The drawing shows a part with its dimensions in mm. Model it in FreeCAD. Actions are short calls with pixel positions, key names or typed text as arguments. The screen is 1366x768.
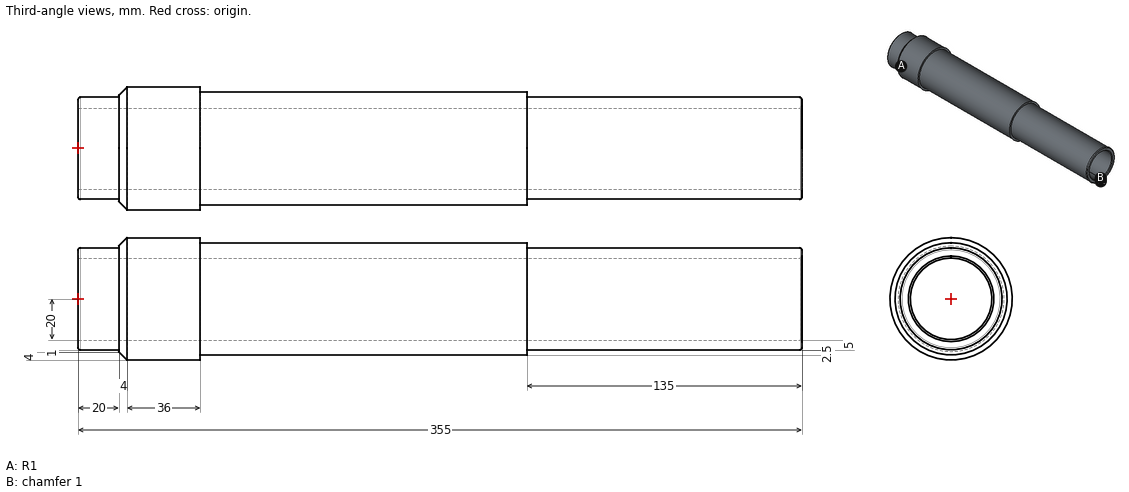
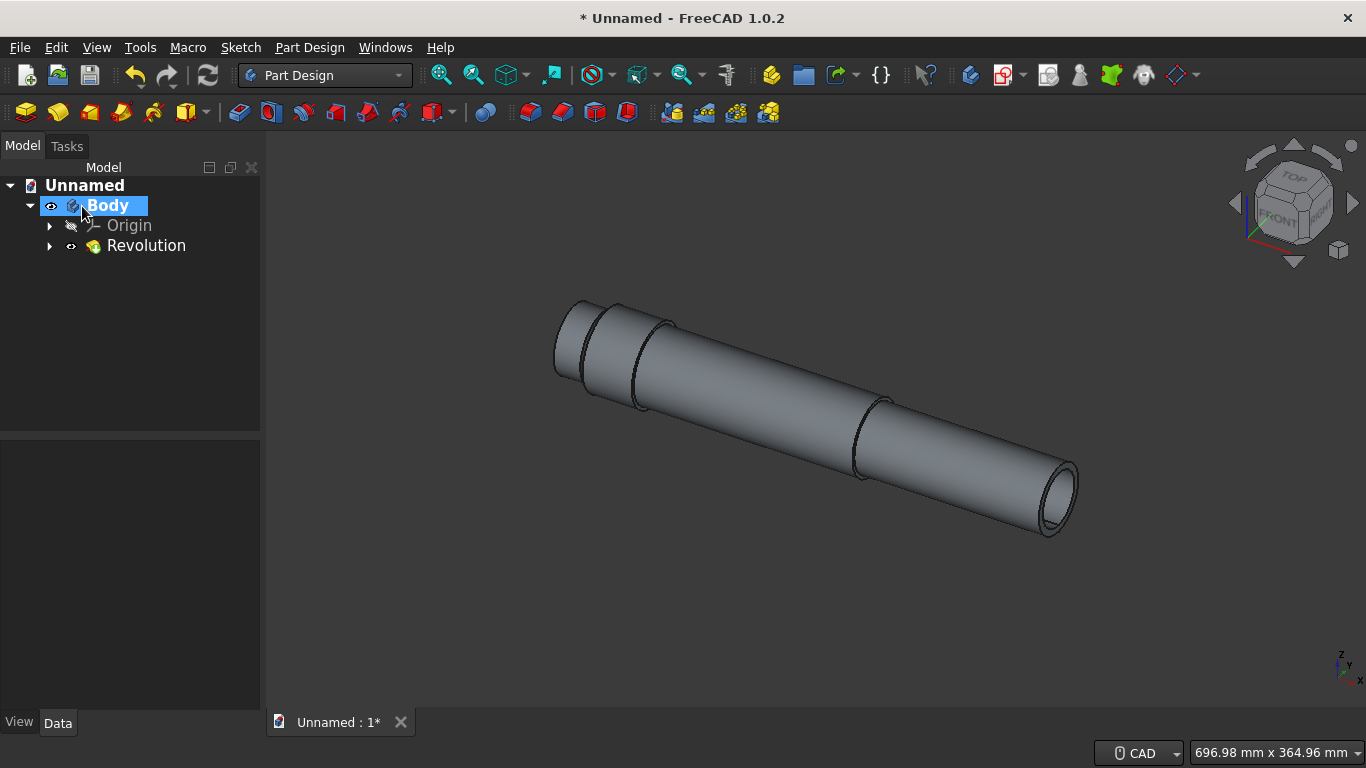
click(1059, 466)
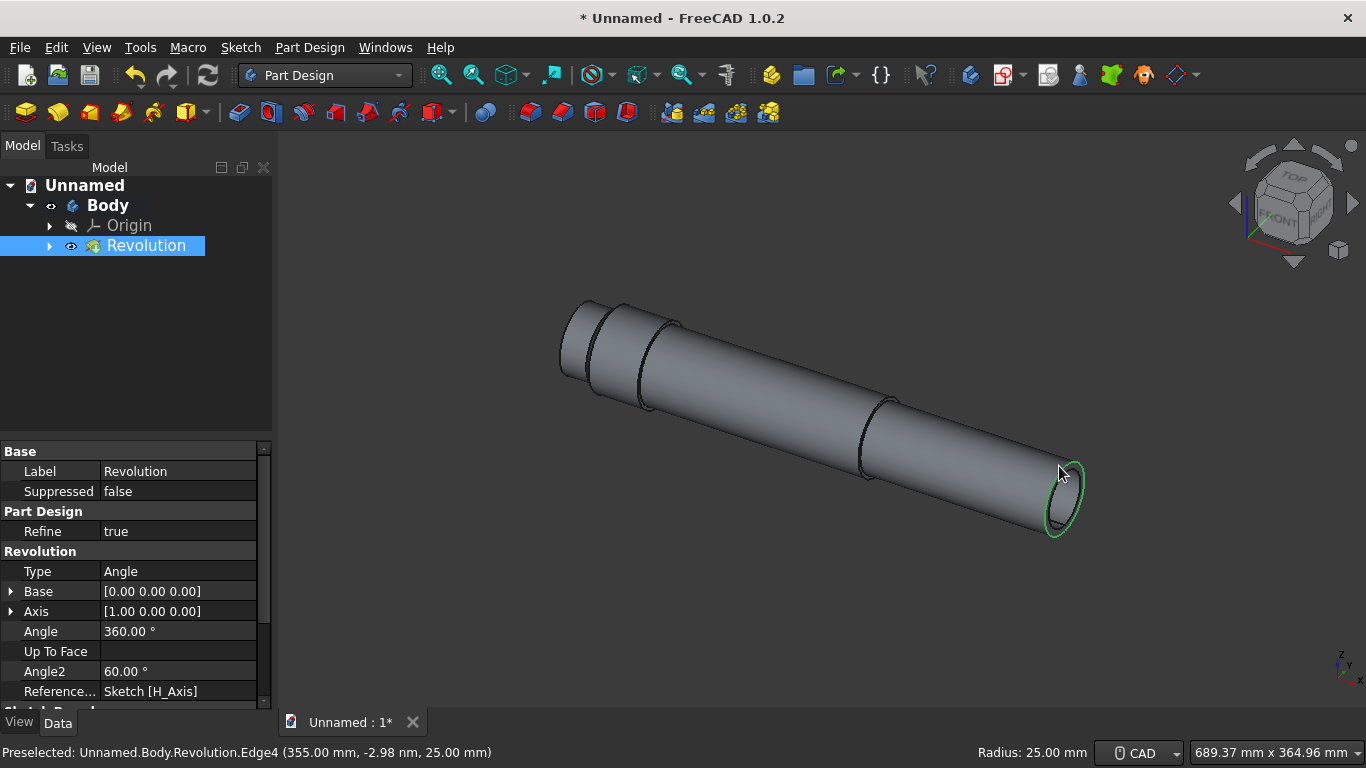
key(0)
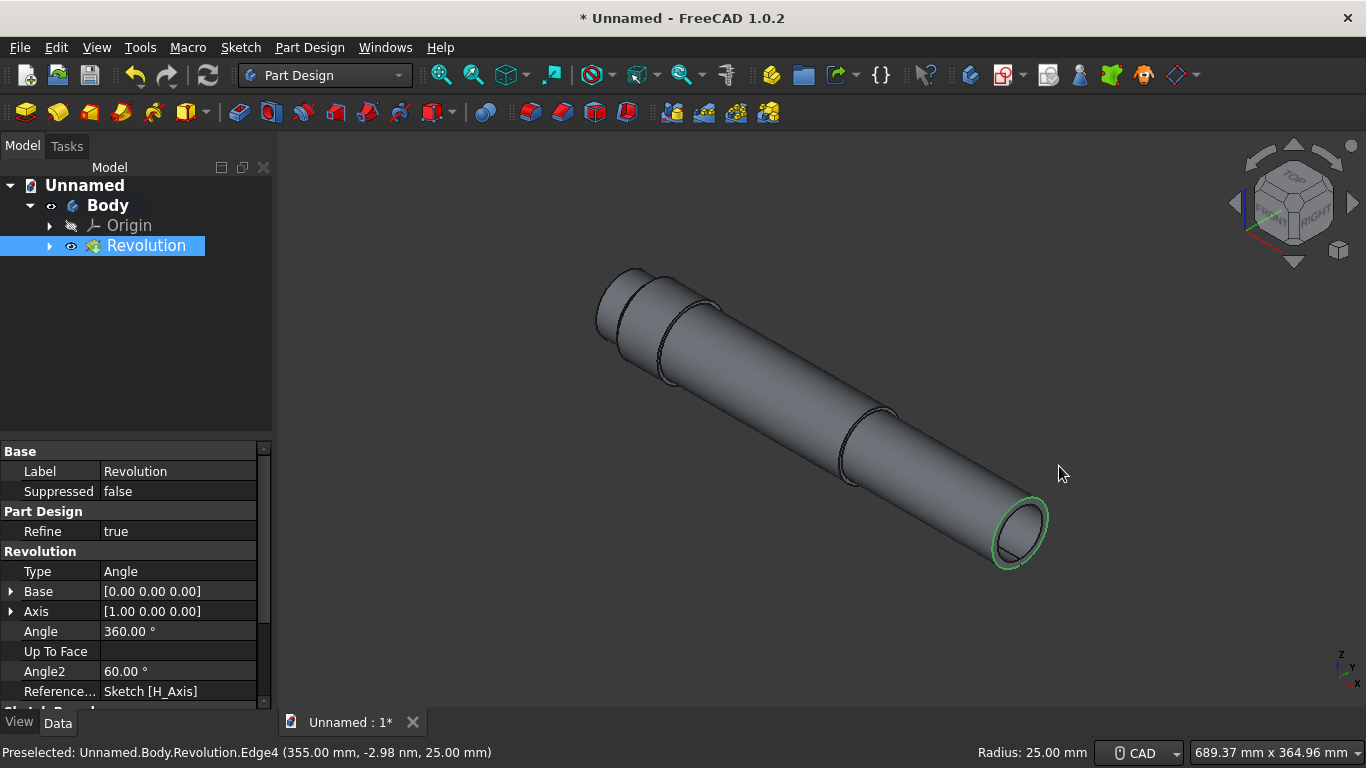
click(597, 329, ctrl)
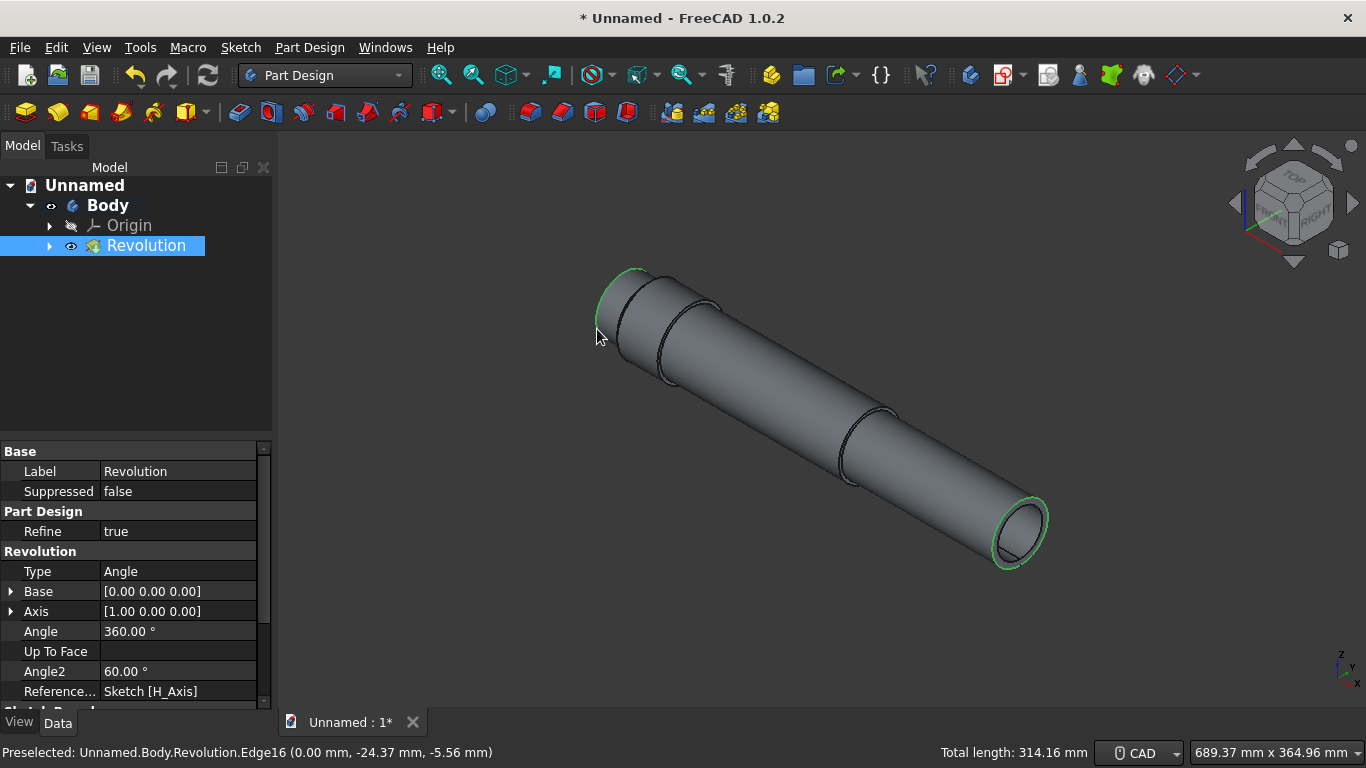
click(532, 112)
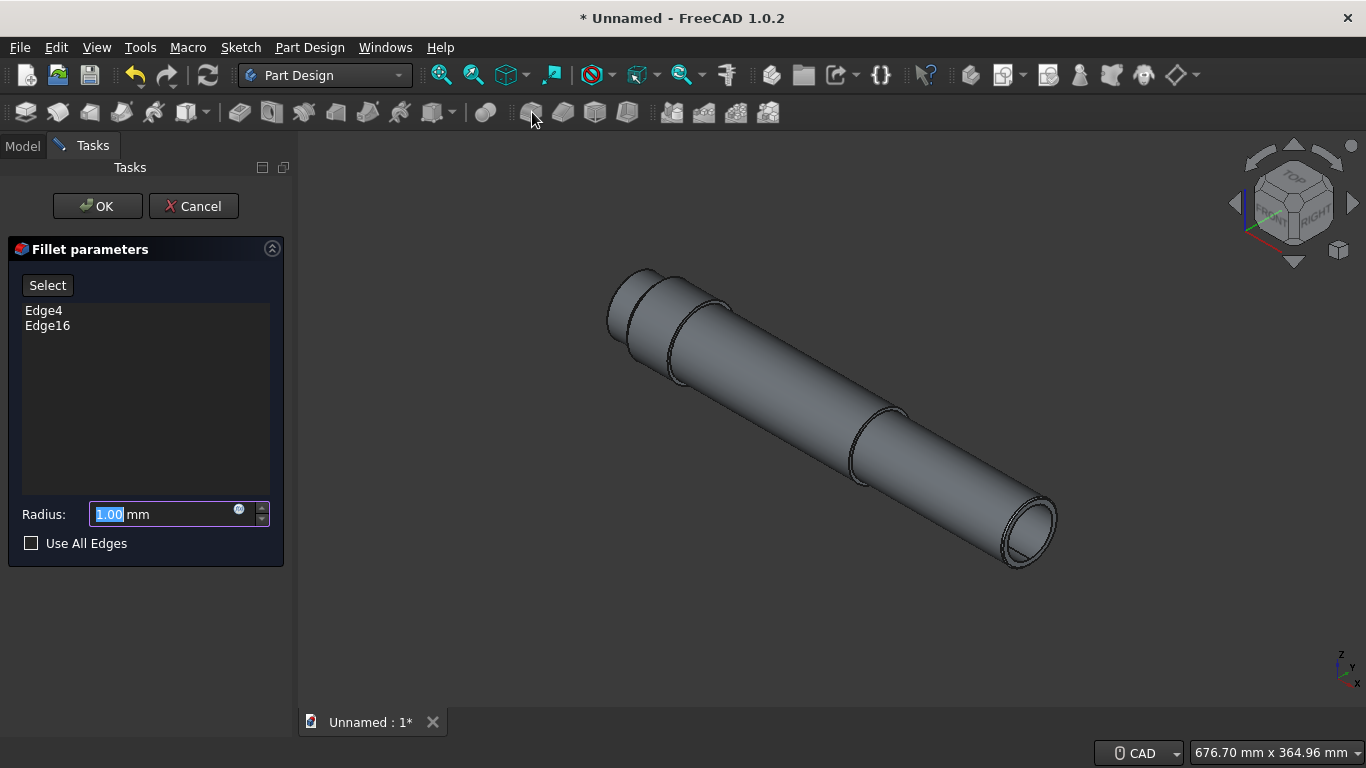
text(1)
key(Tab)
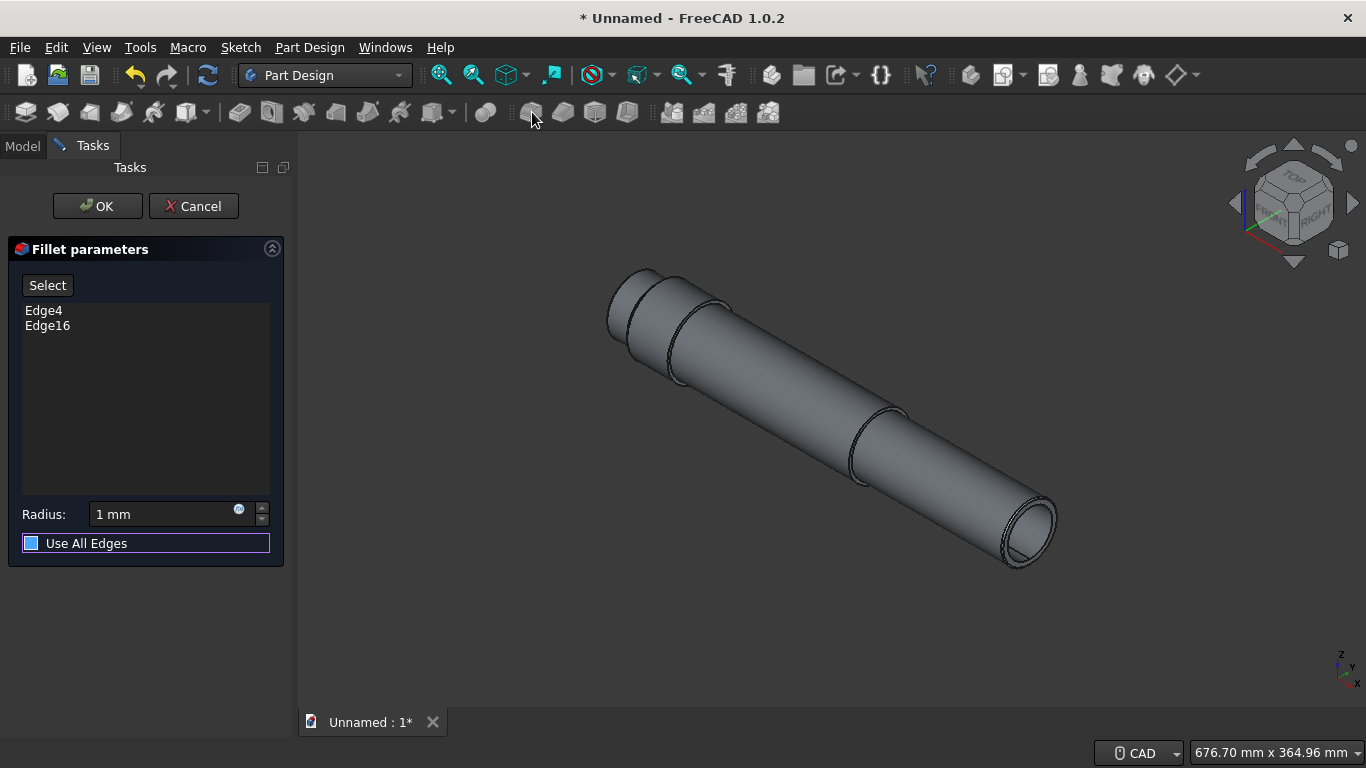
click(98, 206)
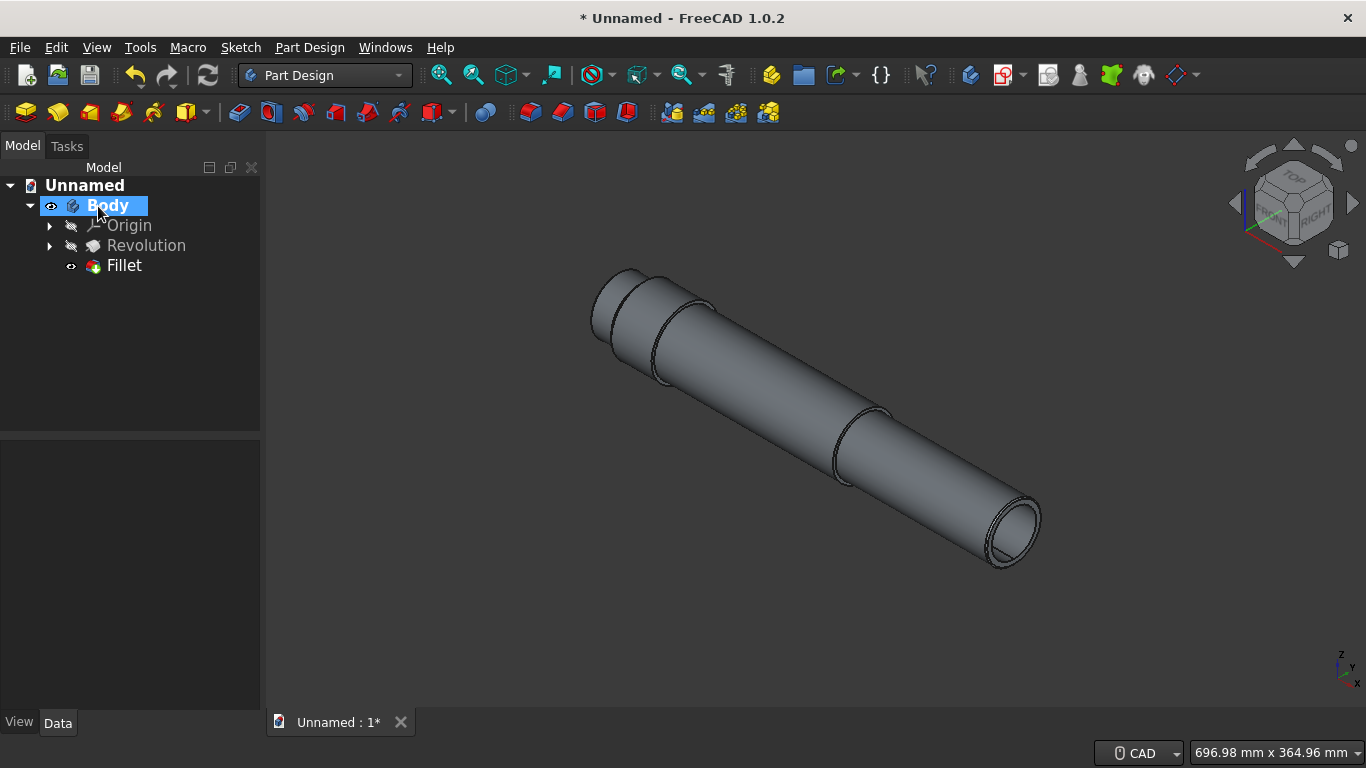
click(1035, 512)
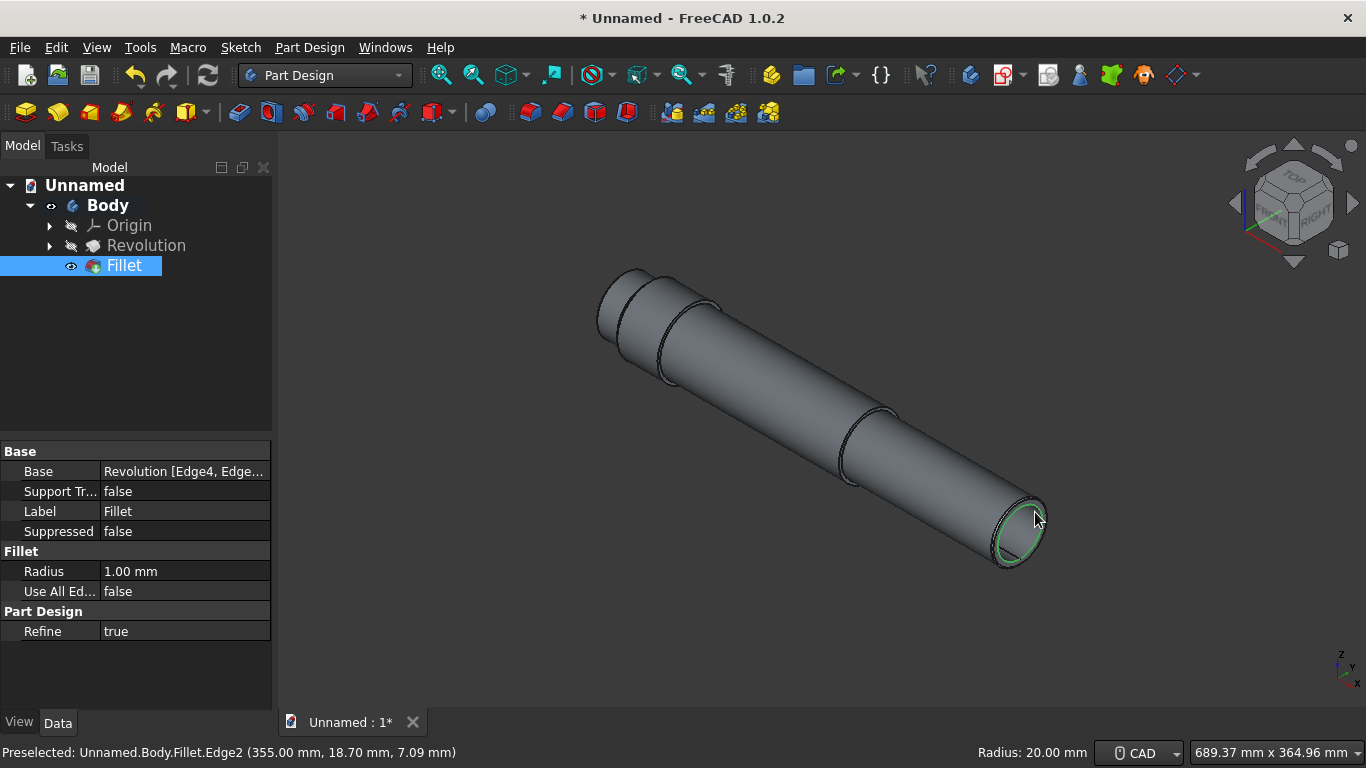
click(564, 112)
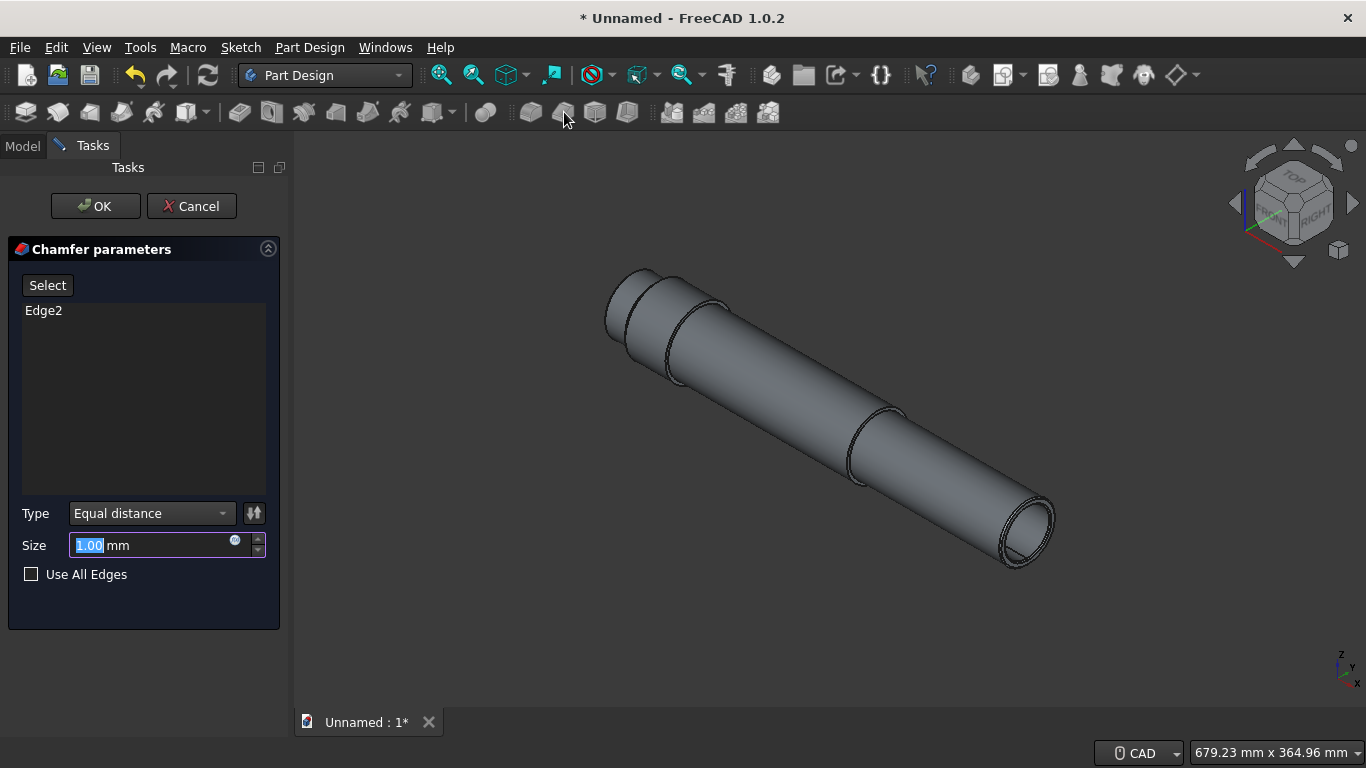
text(1)
key(Tab)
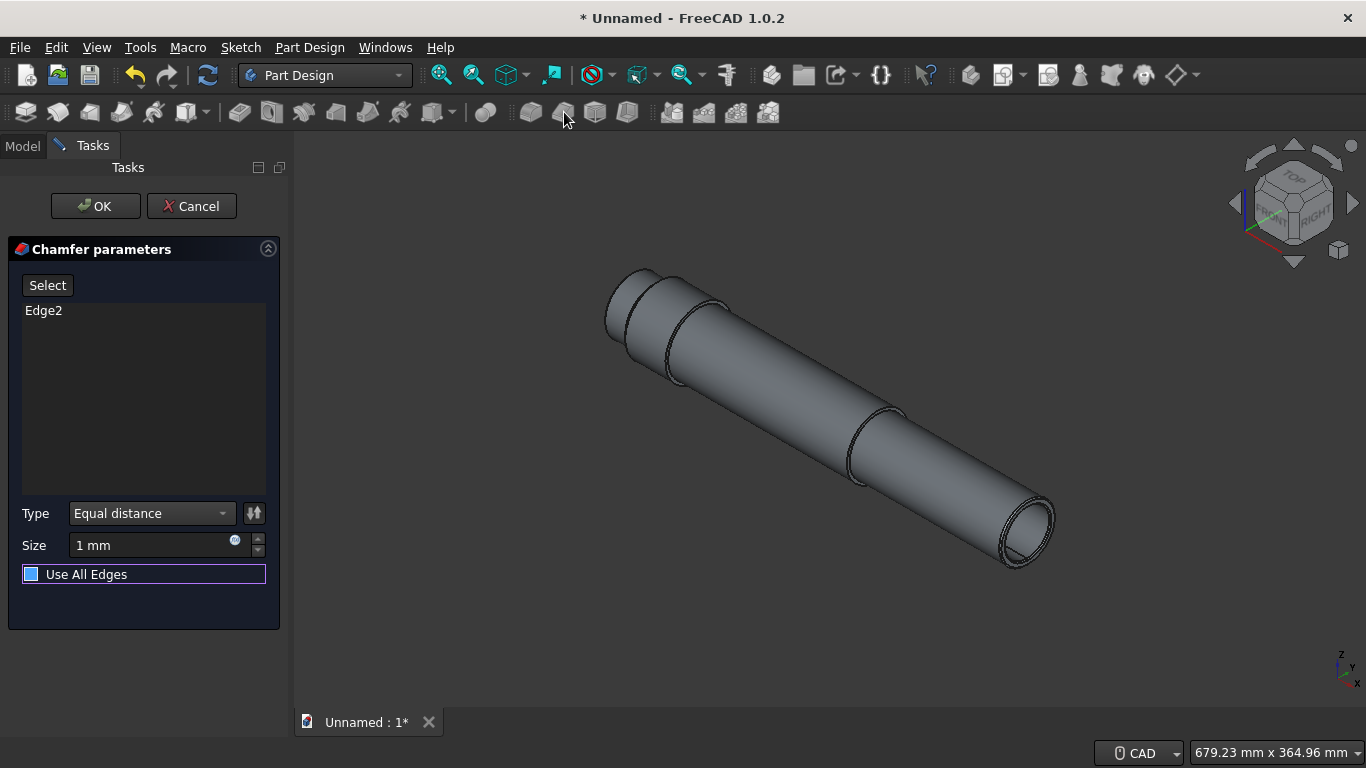
click(96, 206)